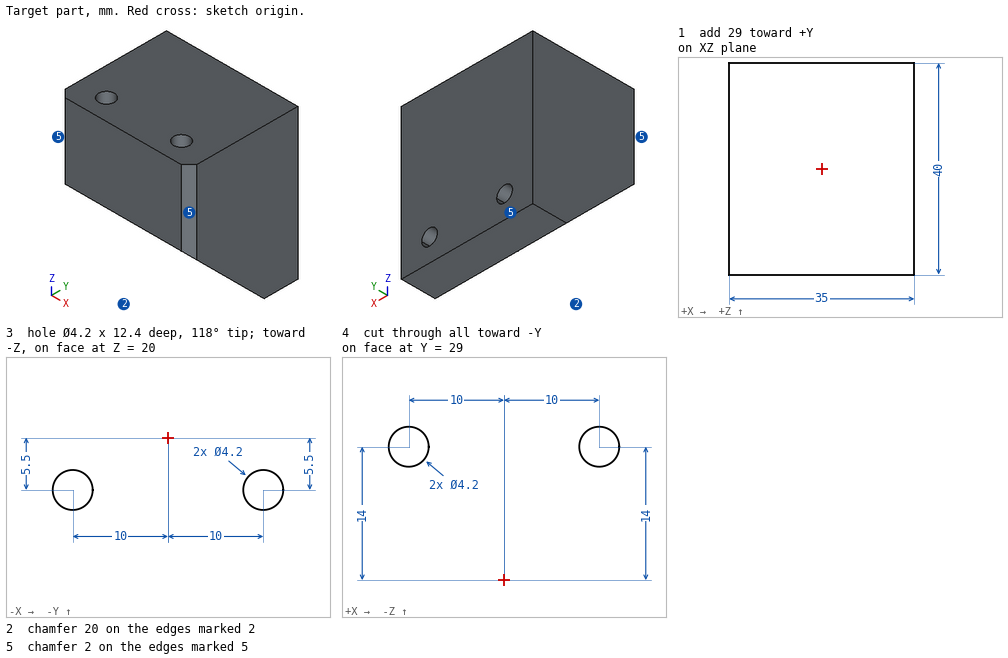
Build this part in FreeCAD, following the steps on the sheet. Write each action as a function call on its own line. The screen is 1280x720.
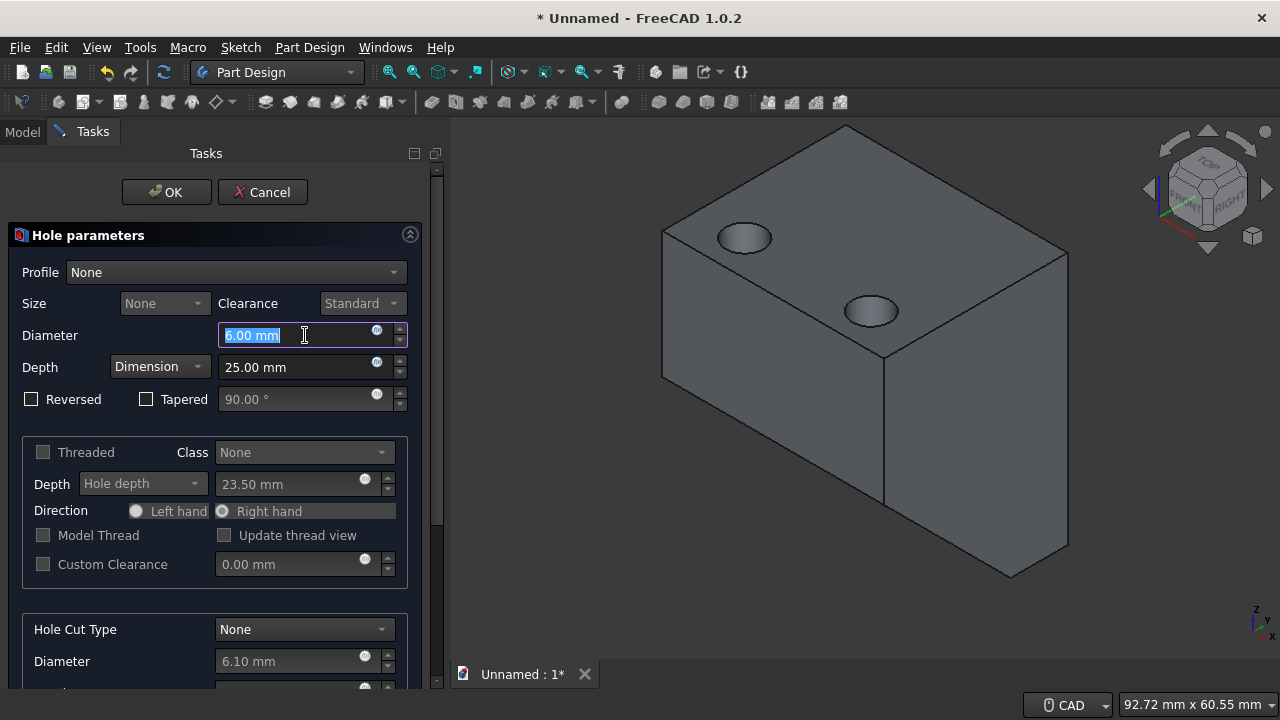
text(4.2)
key(Tab)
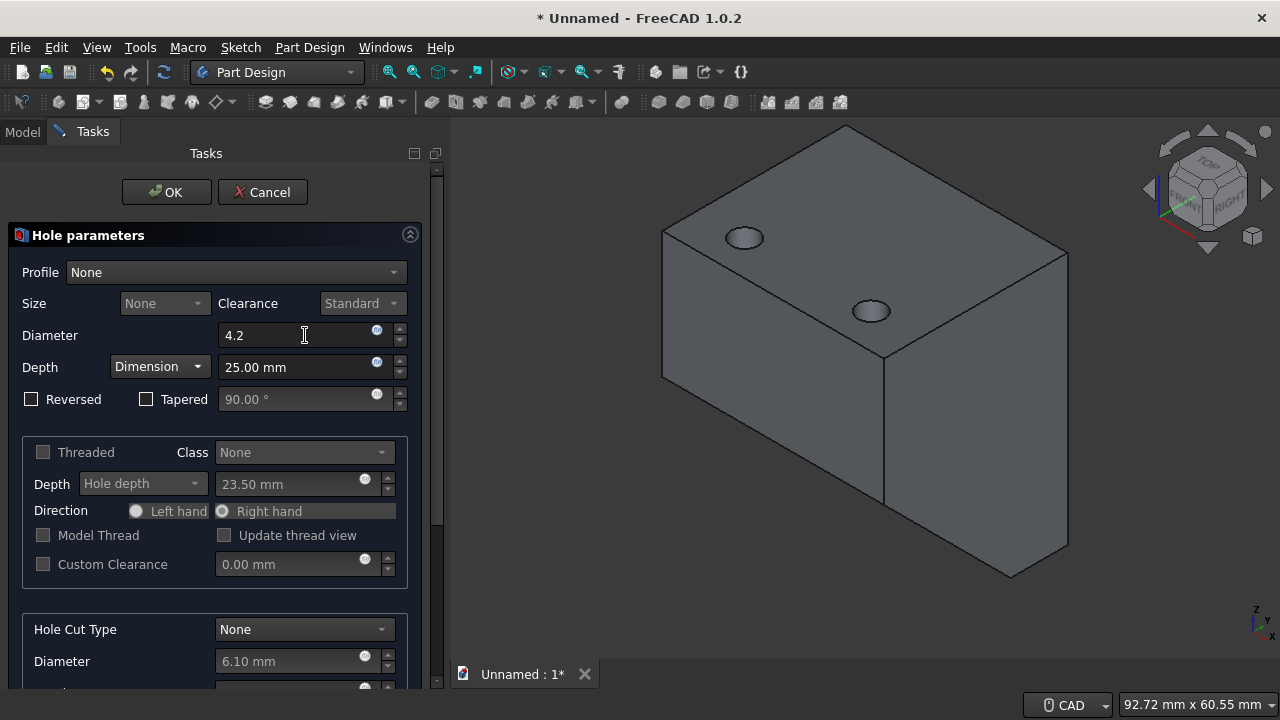
triple_click(305, 367)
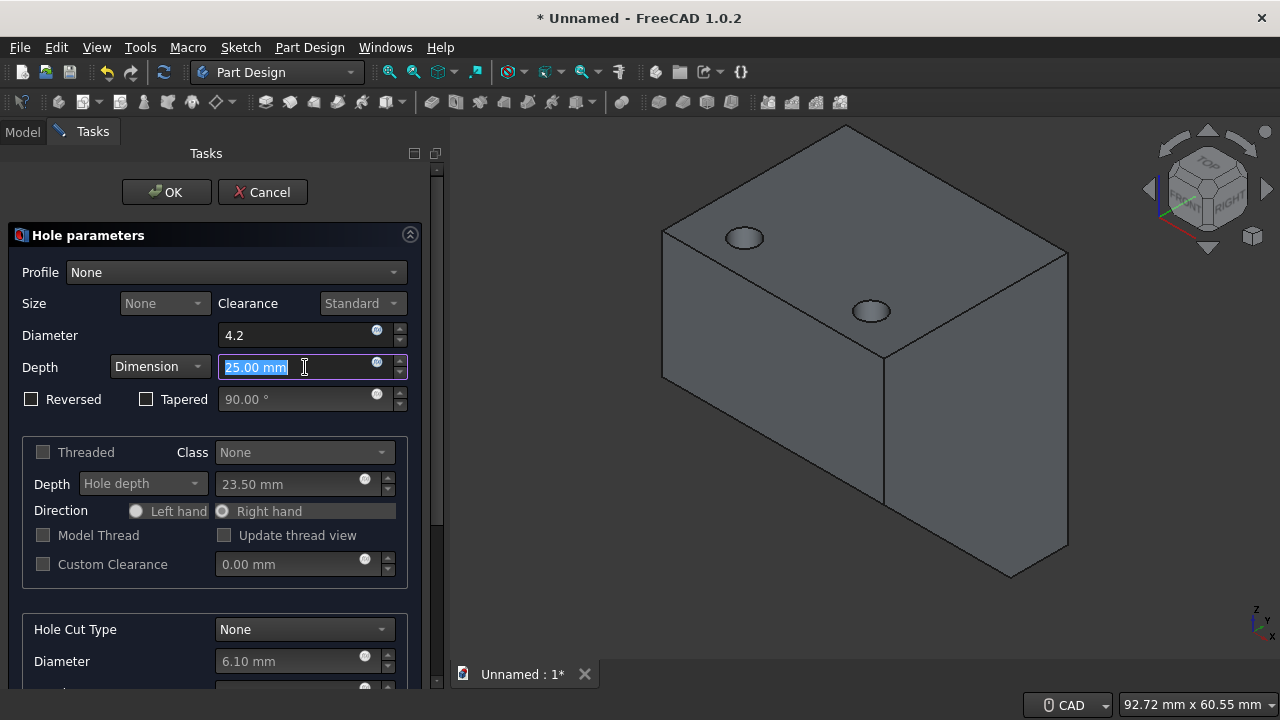
text(12.4)
key(Tab)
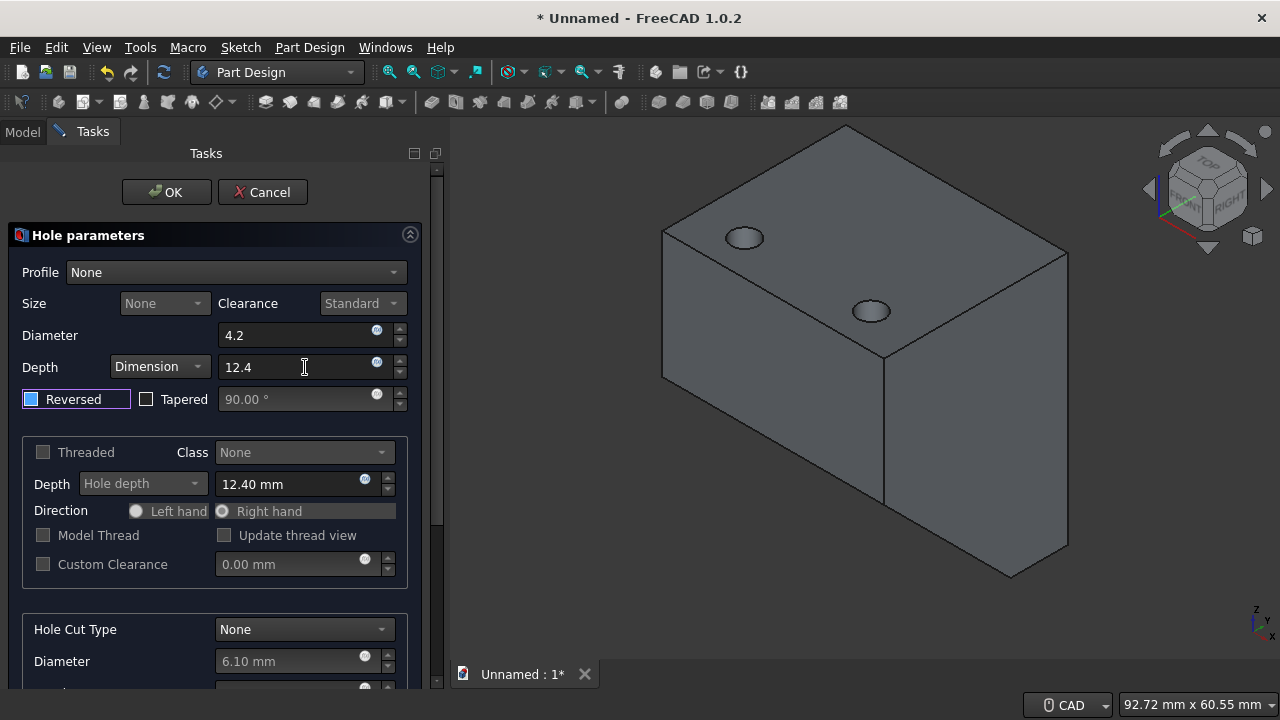
click(167, 192)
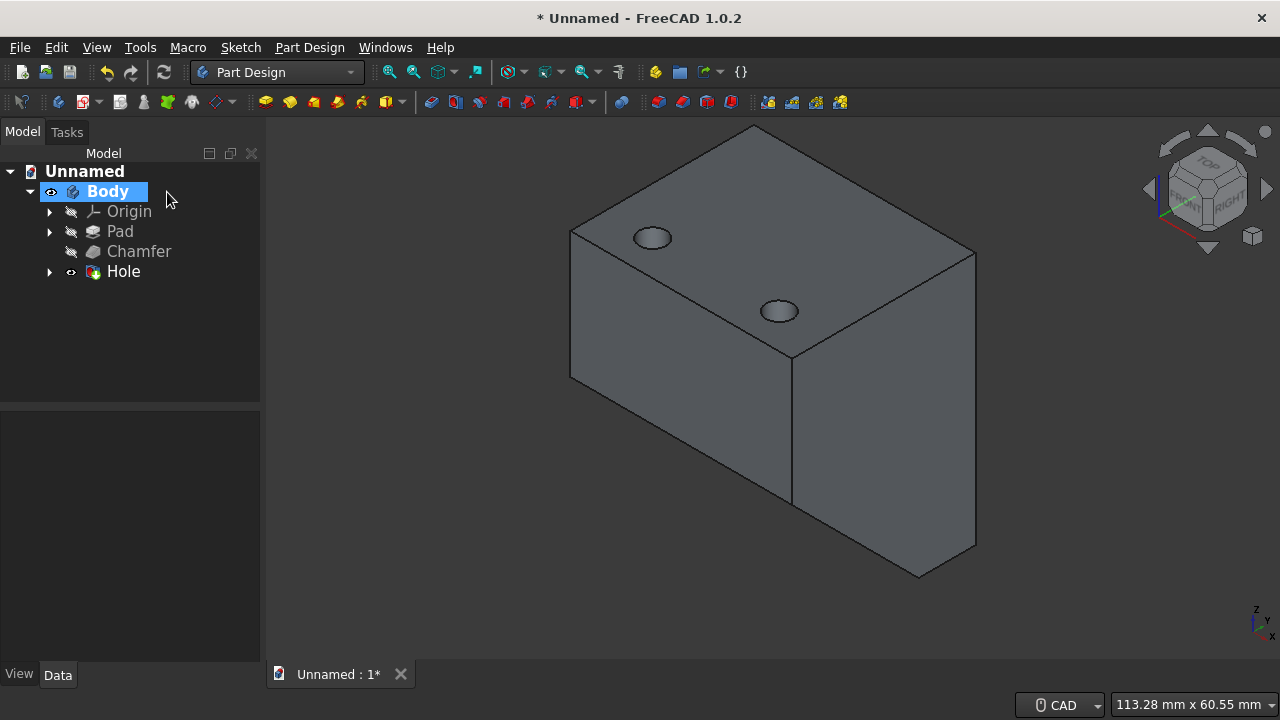
key(4)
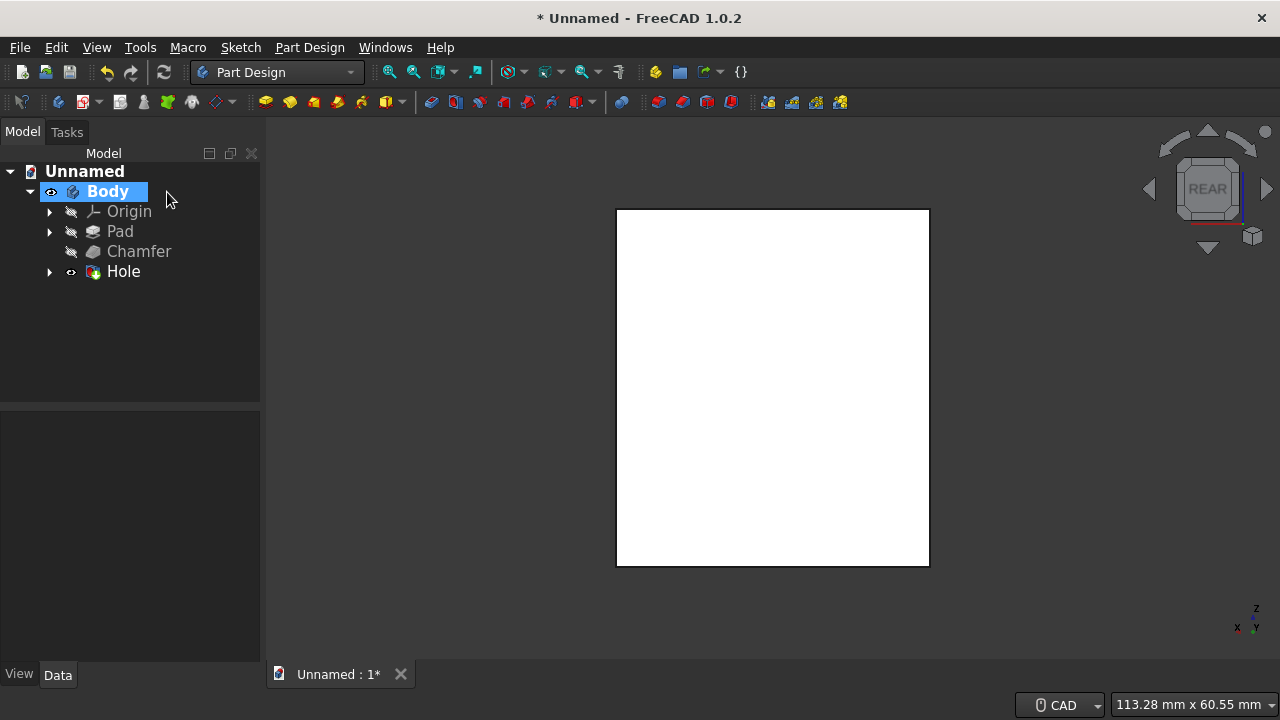
click(773, 387)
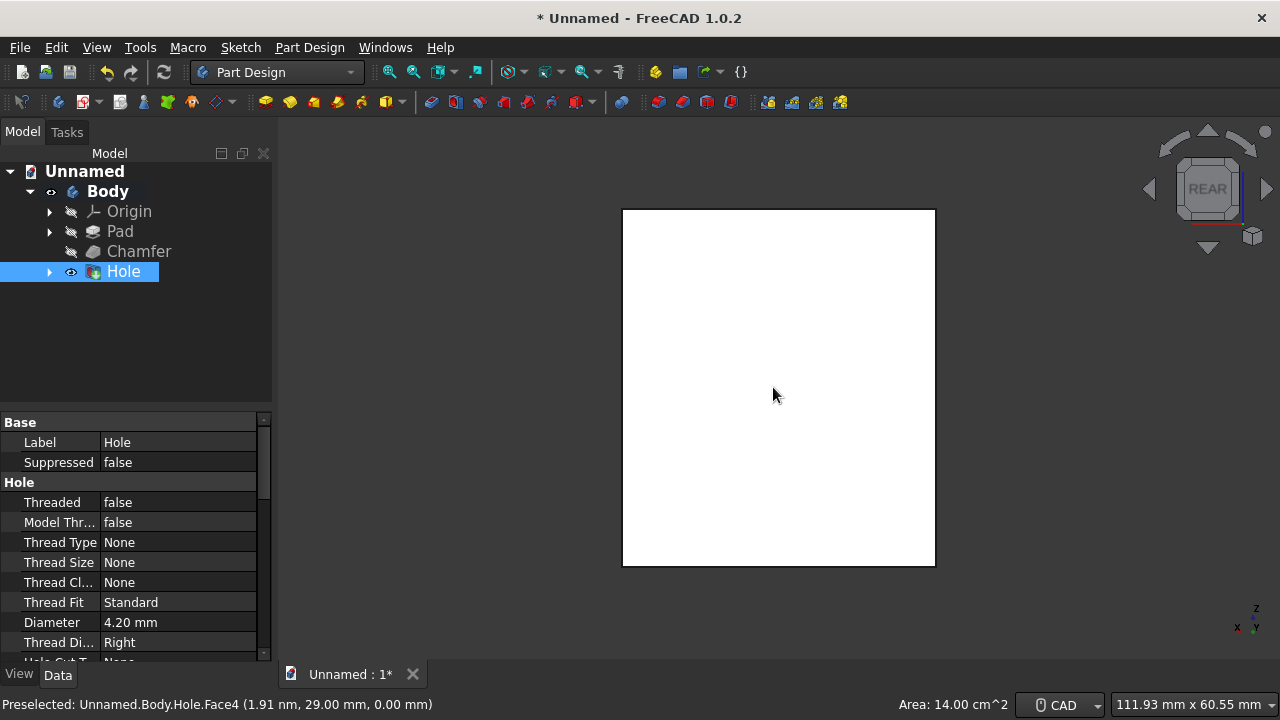
click(84, 102)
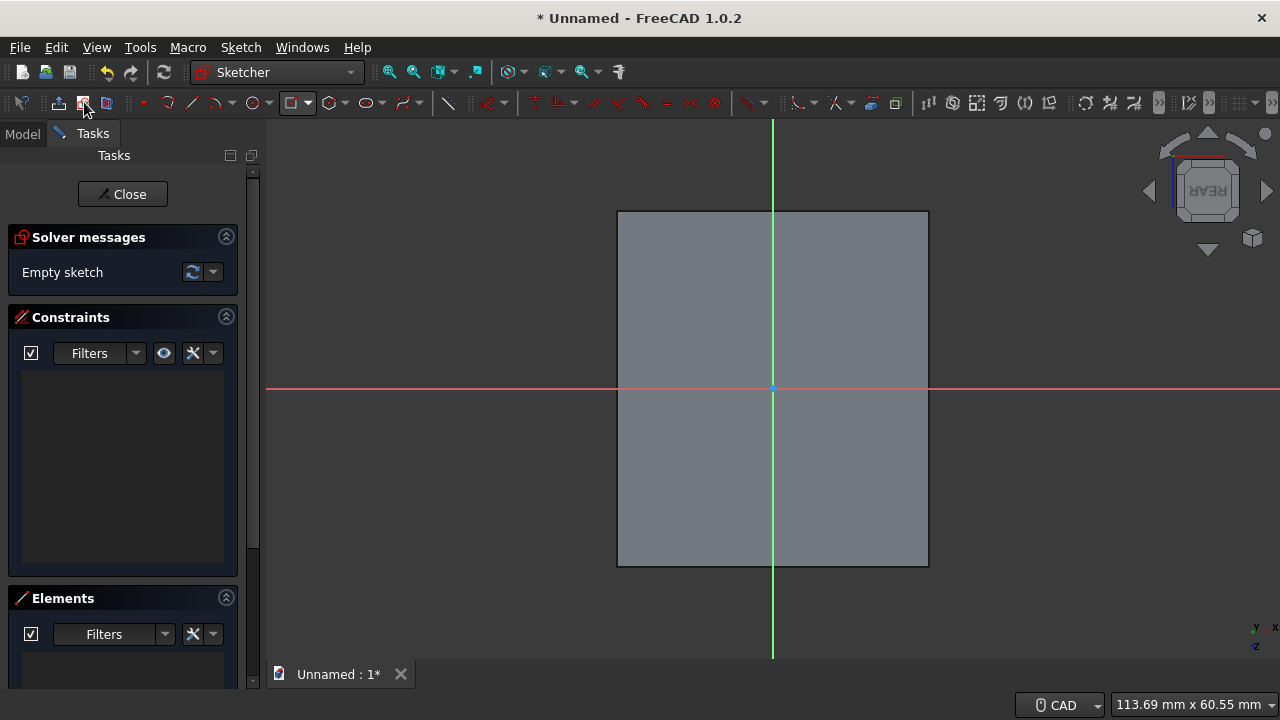
scroll(829, 259, up, 4)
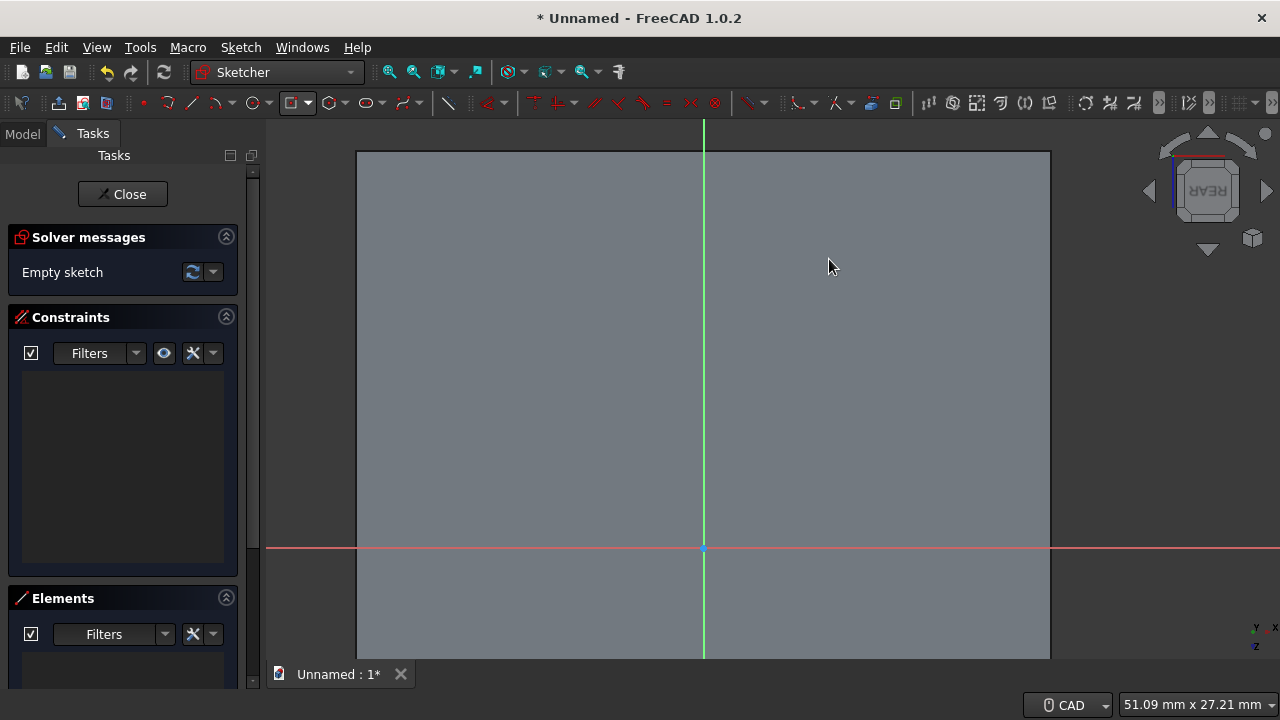
key(g)
key(c)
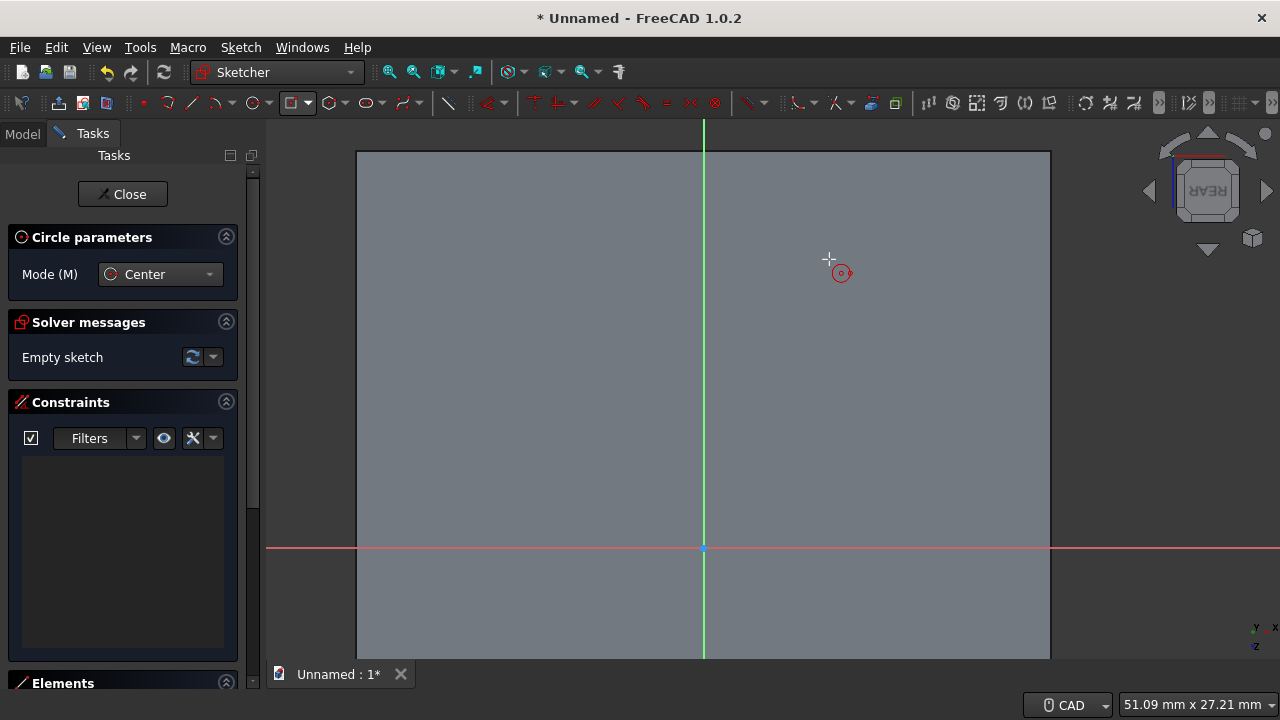
click(505, 270)
move(535, 241)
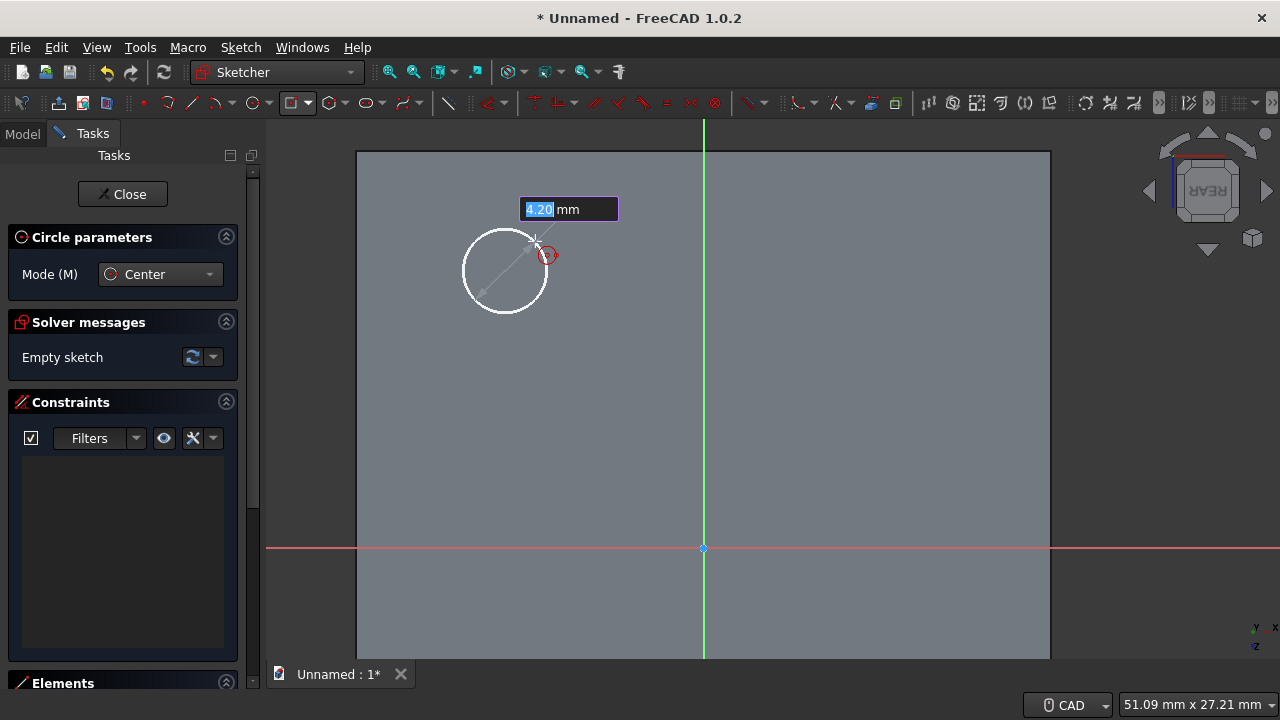
text(4.2)
key(Return)